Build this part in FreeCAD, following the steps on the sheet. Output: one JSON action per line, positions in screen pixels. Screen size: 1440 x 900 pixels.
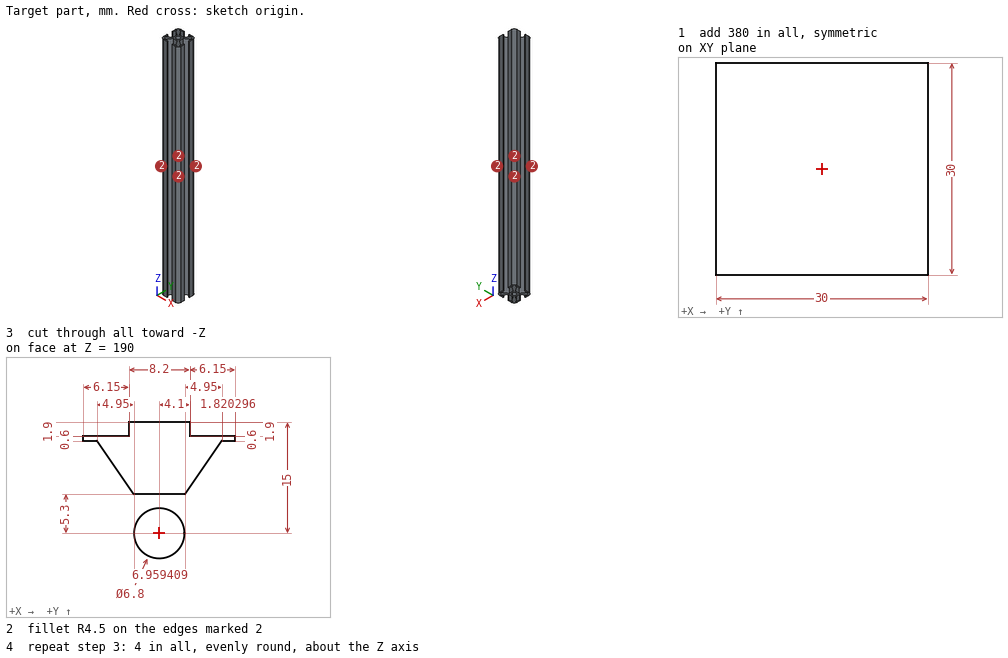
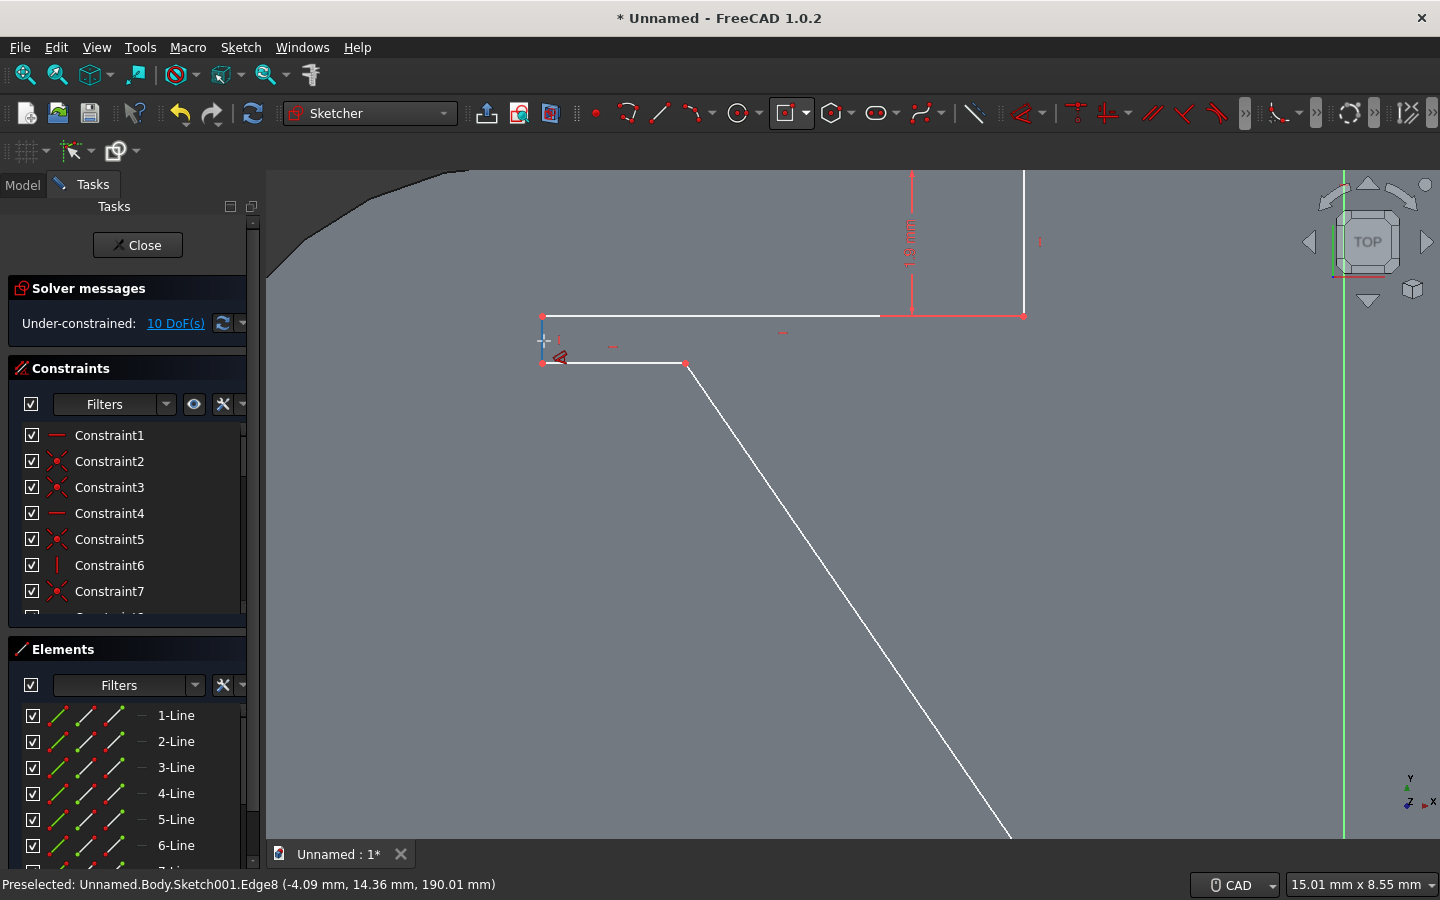
{"action": "left_click", "coordinate": [542, 340]}
{"action": "left_click", "coordinate": [508, 340]}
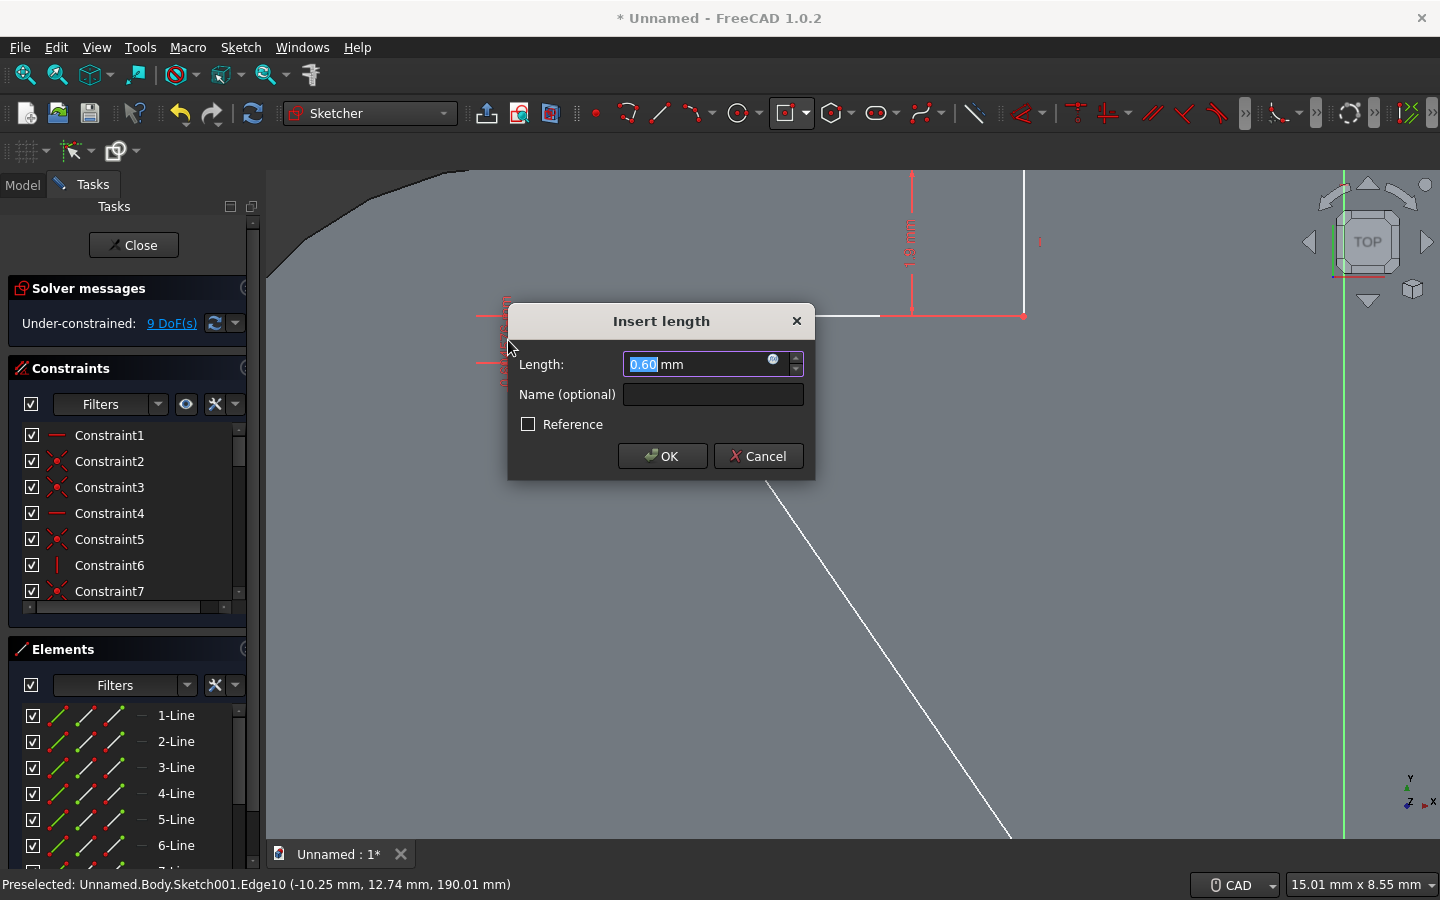
{"action": "type", "text": "0.6"}
{"action": "key", "text": "Return"}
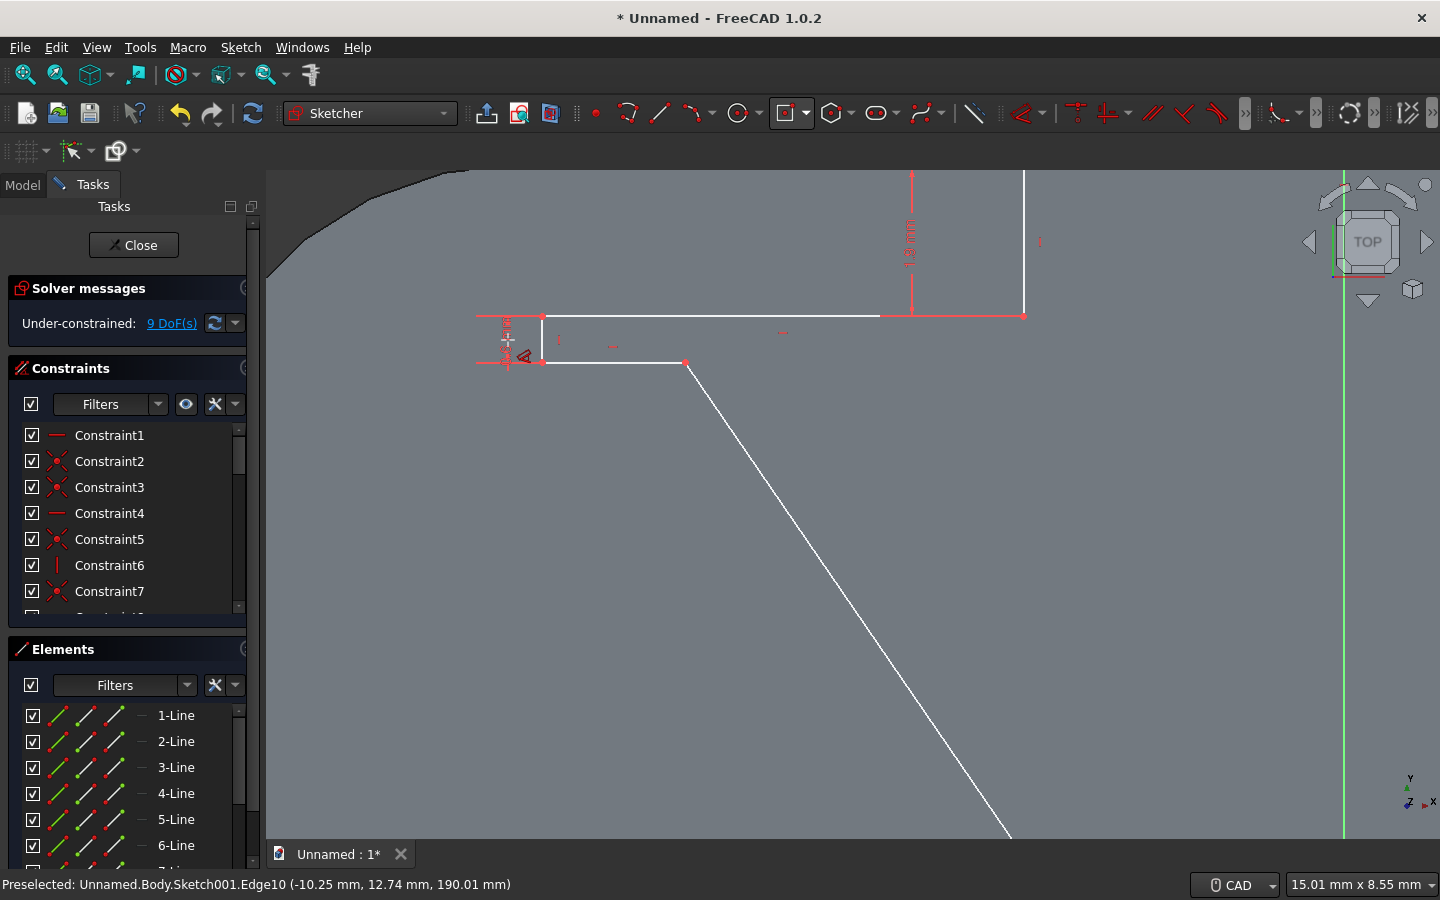
{"action": "scroll", "coordinate": [543, 341], "scroll_direction": "down", "scroll_amount": 6}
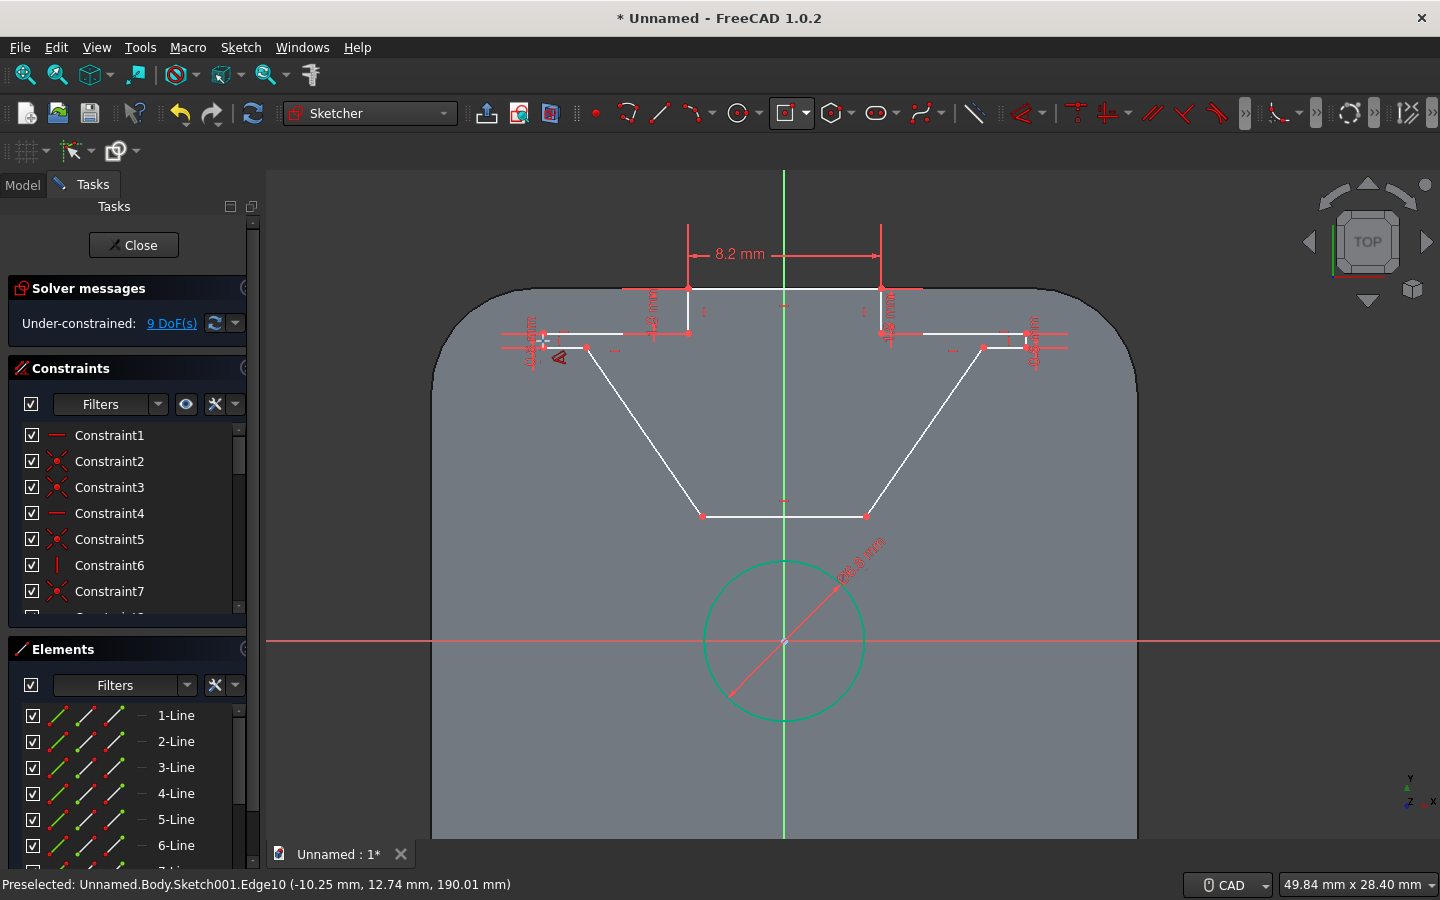
{"action": "left_click", "coordinate": [881, 289]}
{"action": "left_click", "coordinate": [915, 384]}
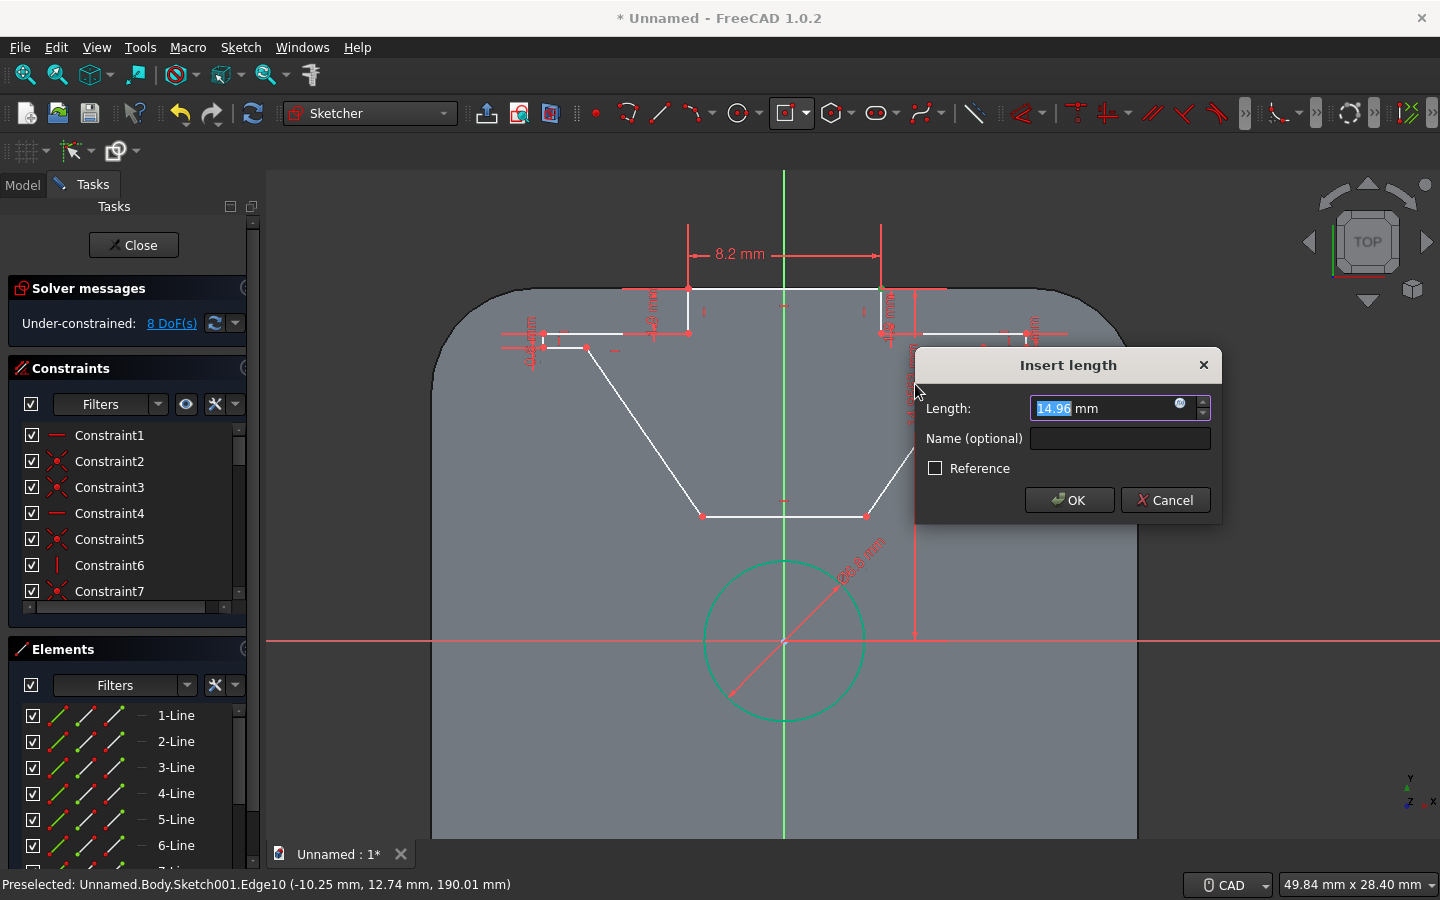
{"action": "type", "text": "15"}
{"action": "key", "text": "Return"}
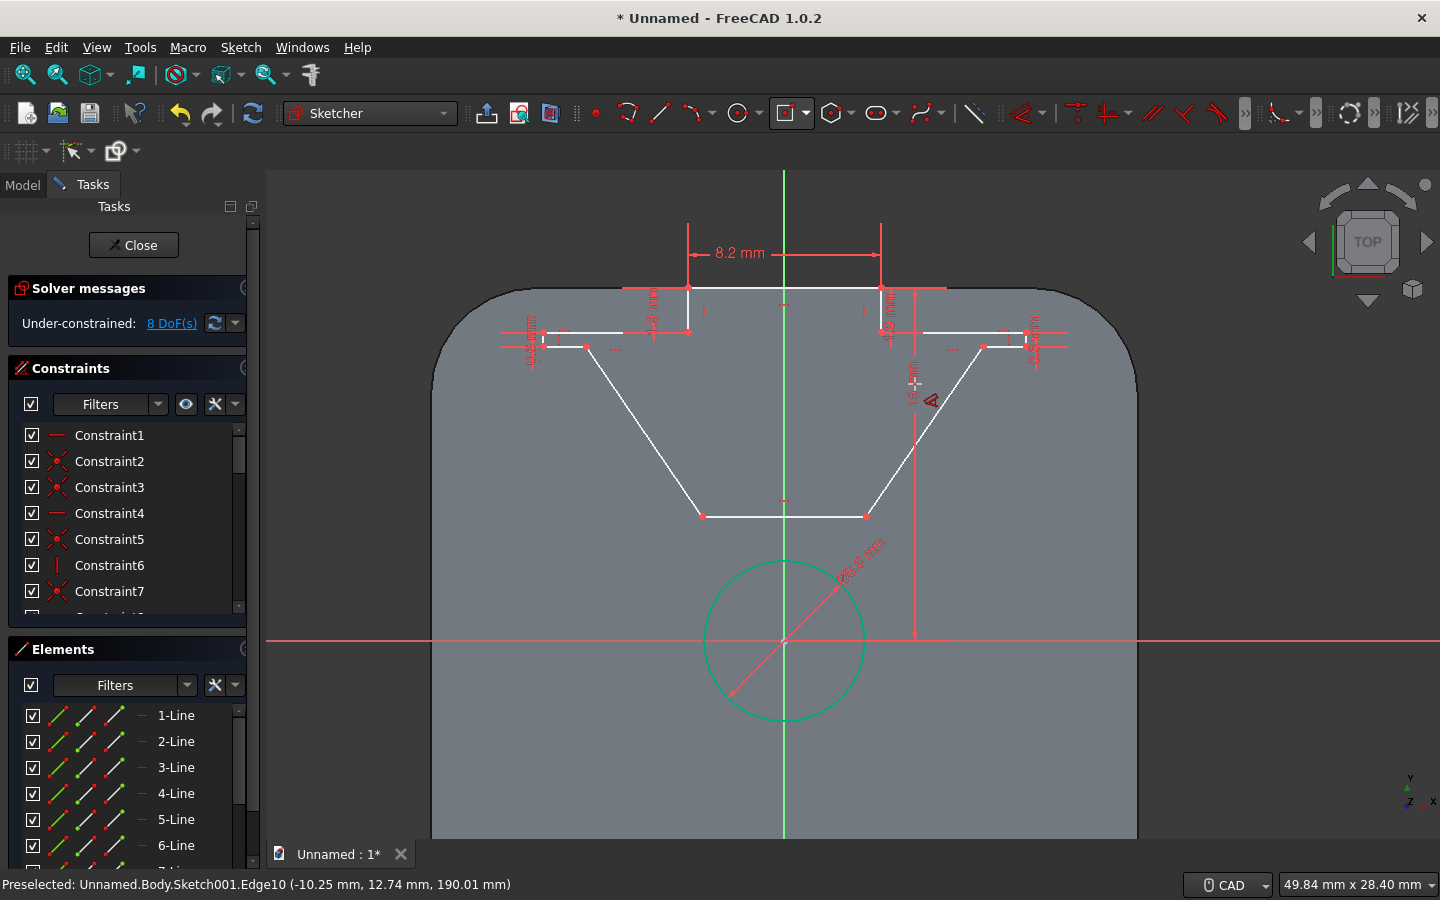
{"action": "left_click", "coordinate": [983, 333]}
{"action": "left_click", "coordinate": [987, 299]}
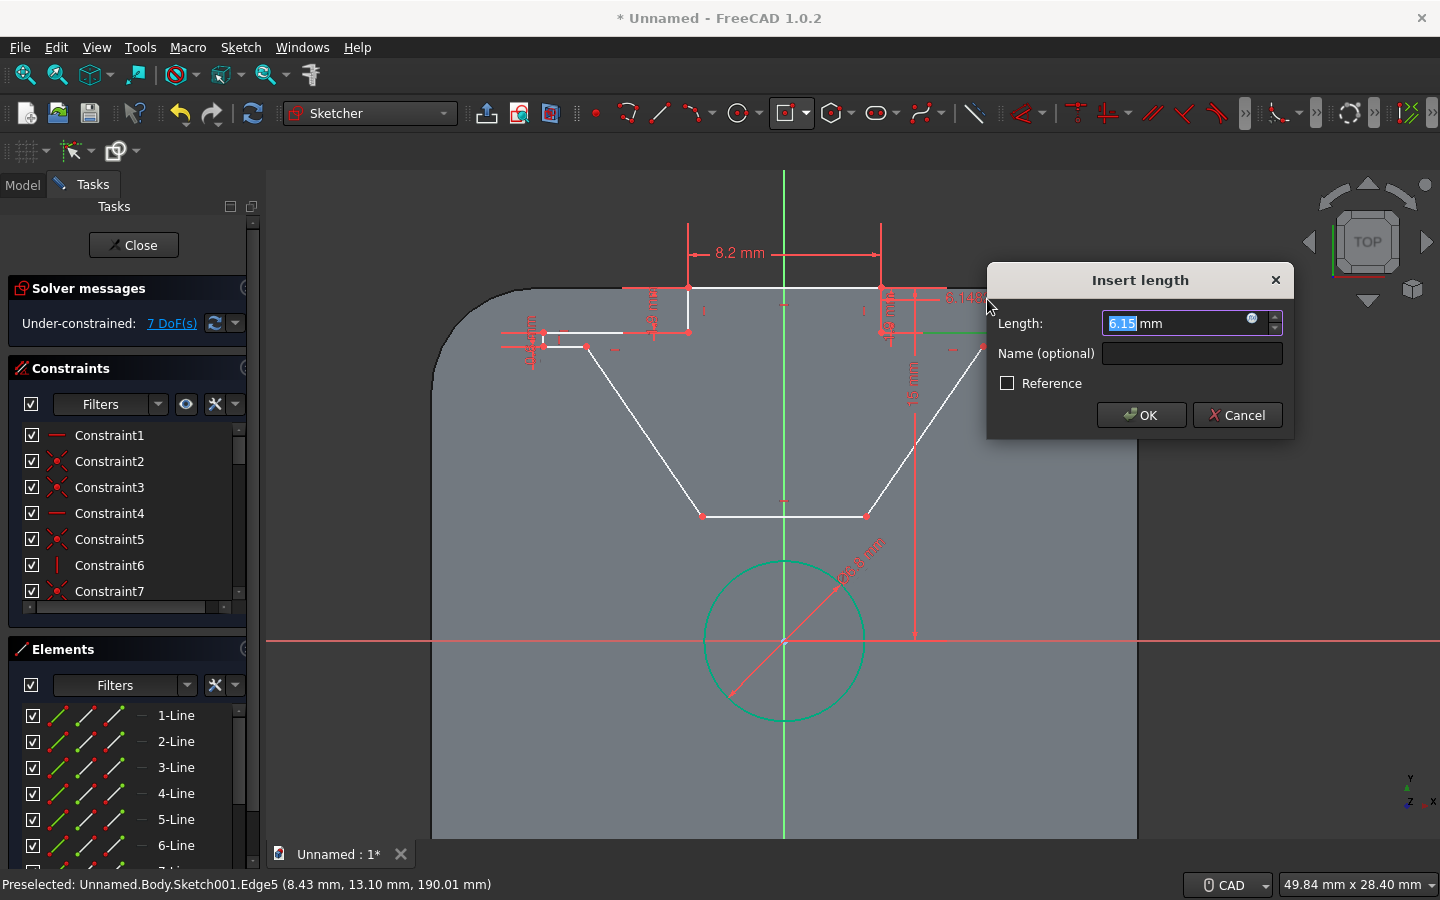
{"action": "type", "text": "6.15"}
{"action": "key", "text": "Return"}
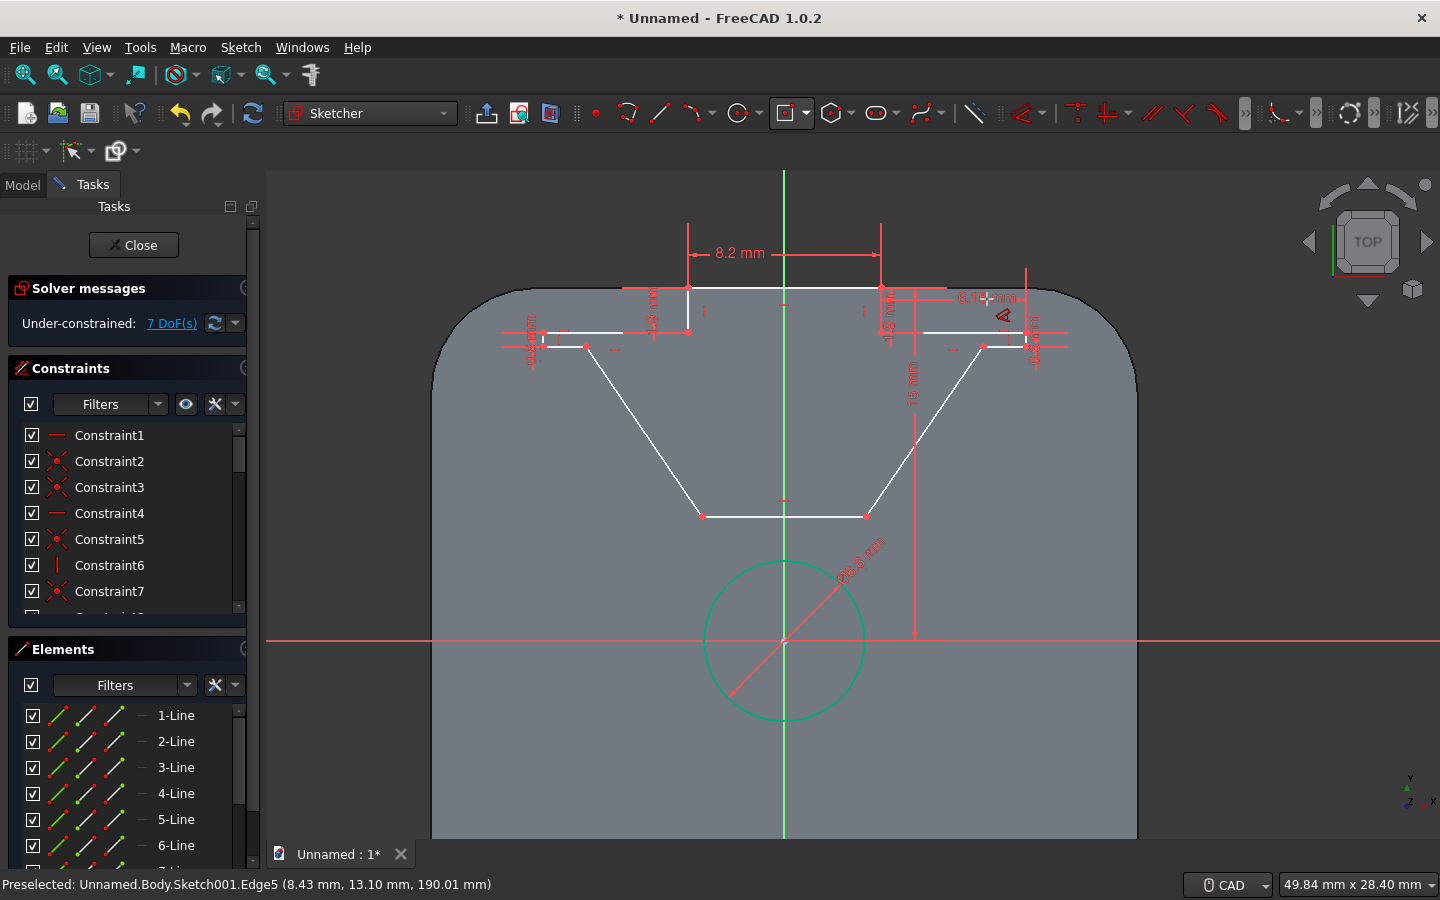
{"action": "left_click", "coordinate": [645, 333]}
{"action": "left_click", "coordinate": [582, 299]}